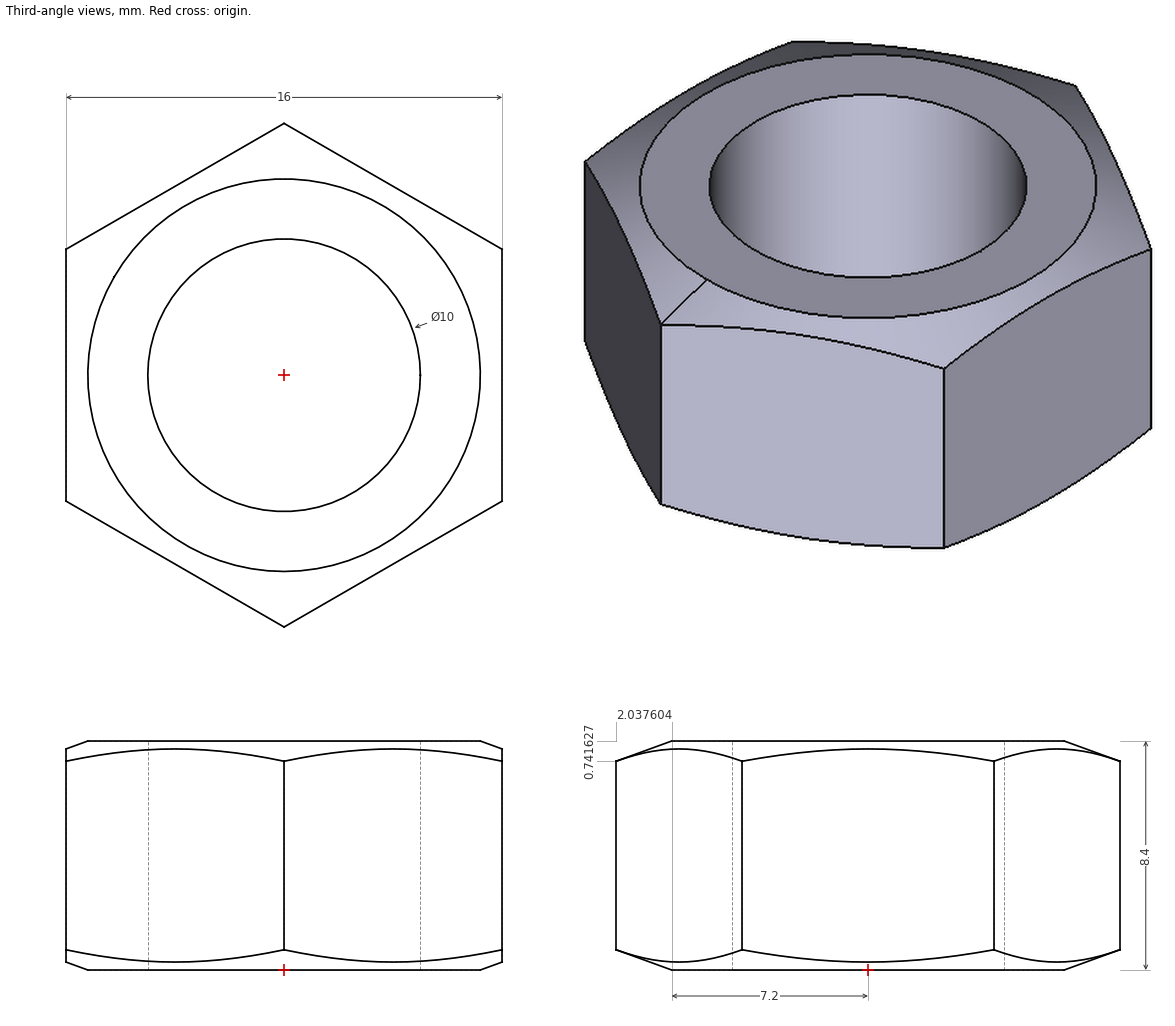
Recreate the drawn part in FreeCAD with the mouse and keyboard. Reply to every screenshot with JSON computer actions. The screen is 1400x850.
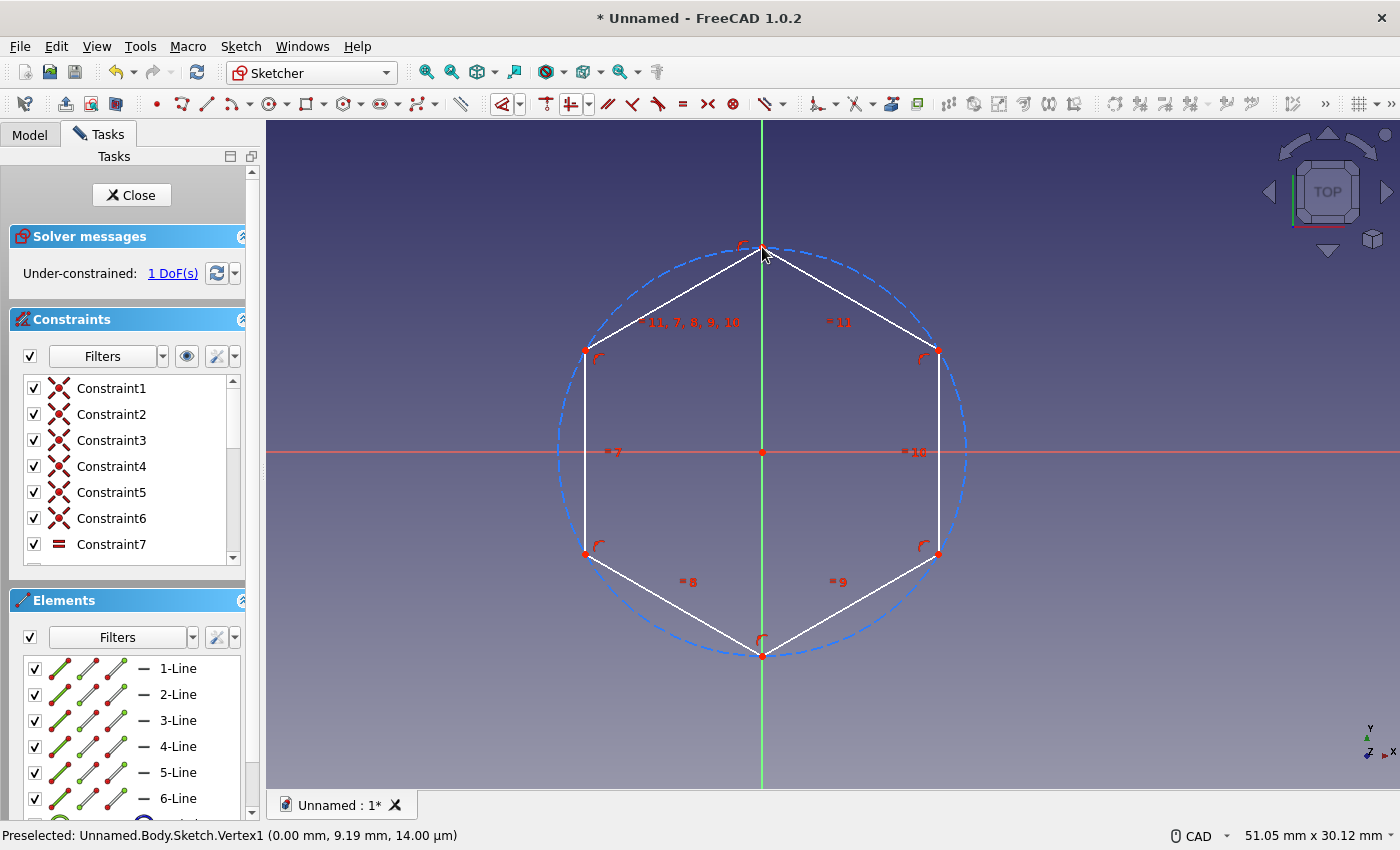
{"action": "left_click", "coordinate": [585, 350]}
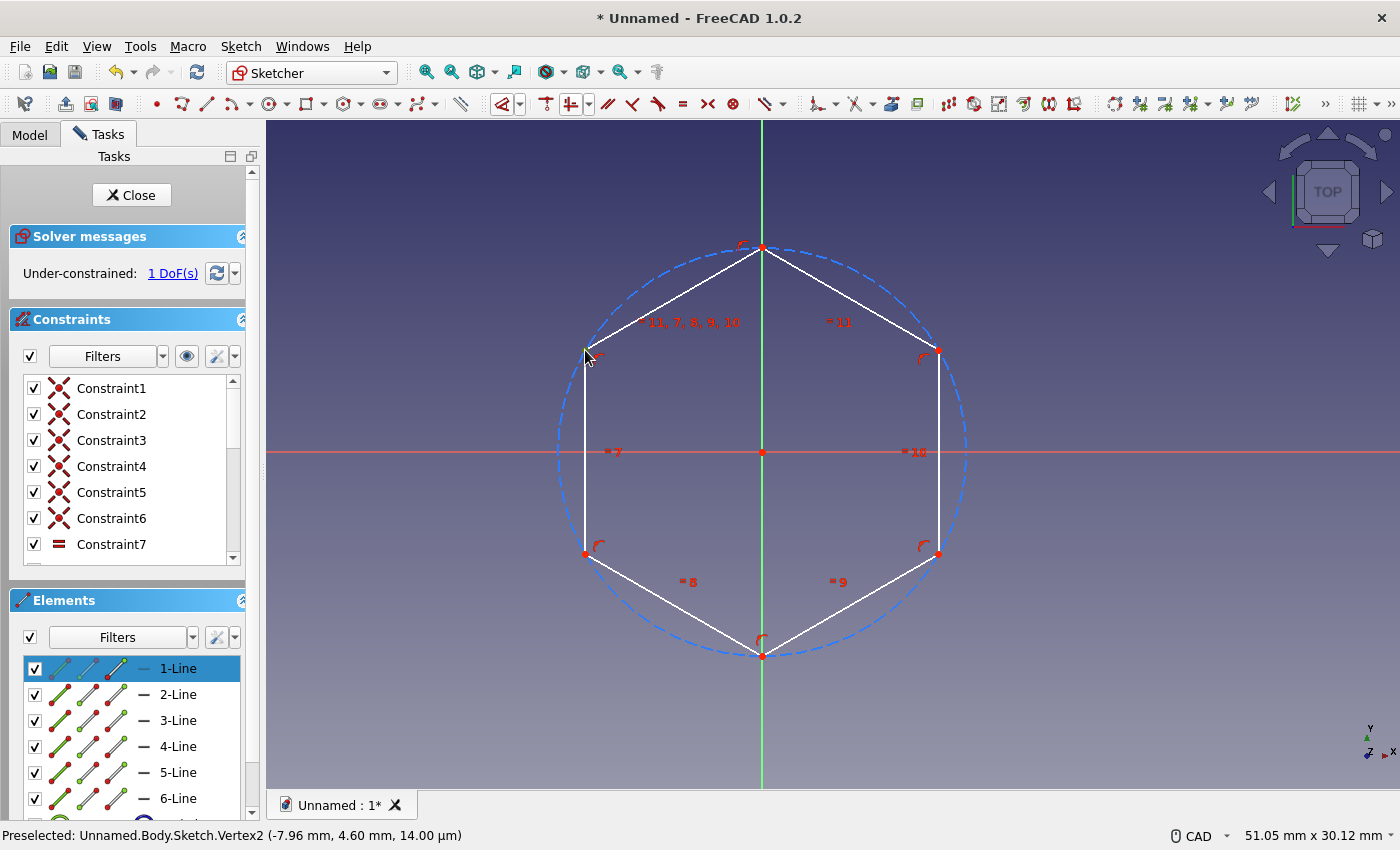
{"action": "left_click", "coordinate": [939, 554]}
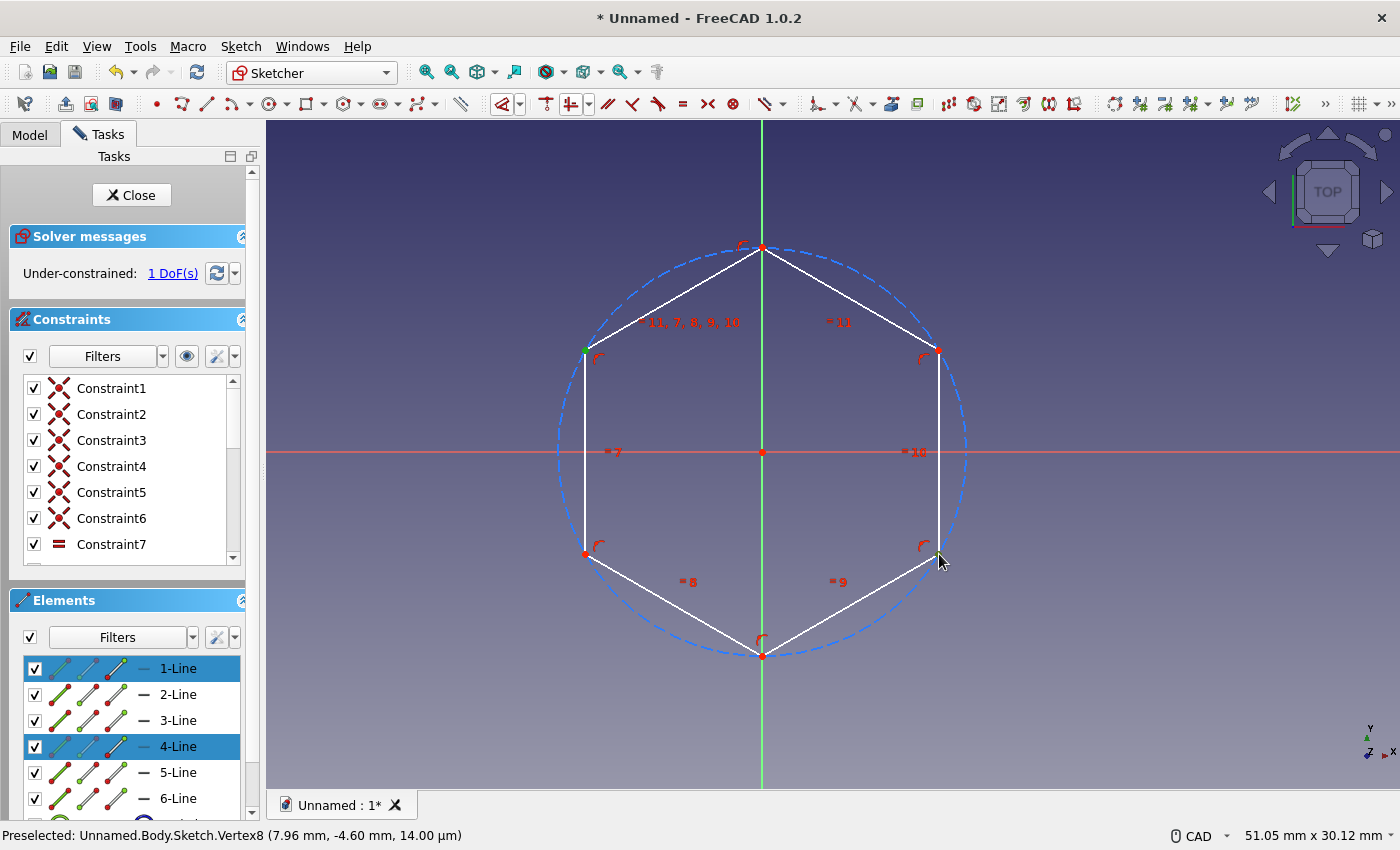
{"action": "left_click", "coordinate": [520, 104]}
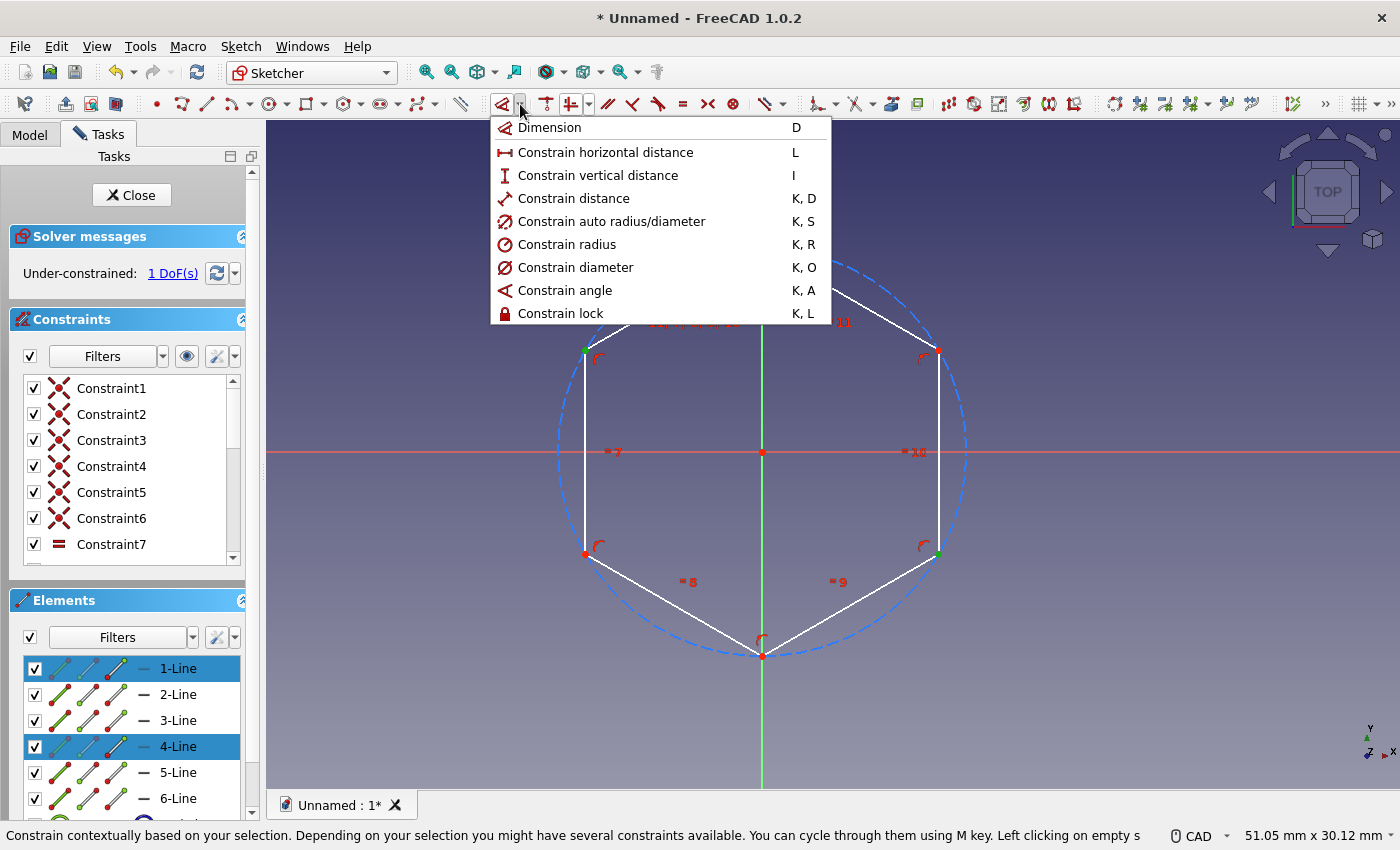
{"action": "left_click", "coordinate": [661, 152]}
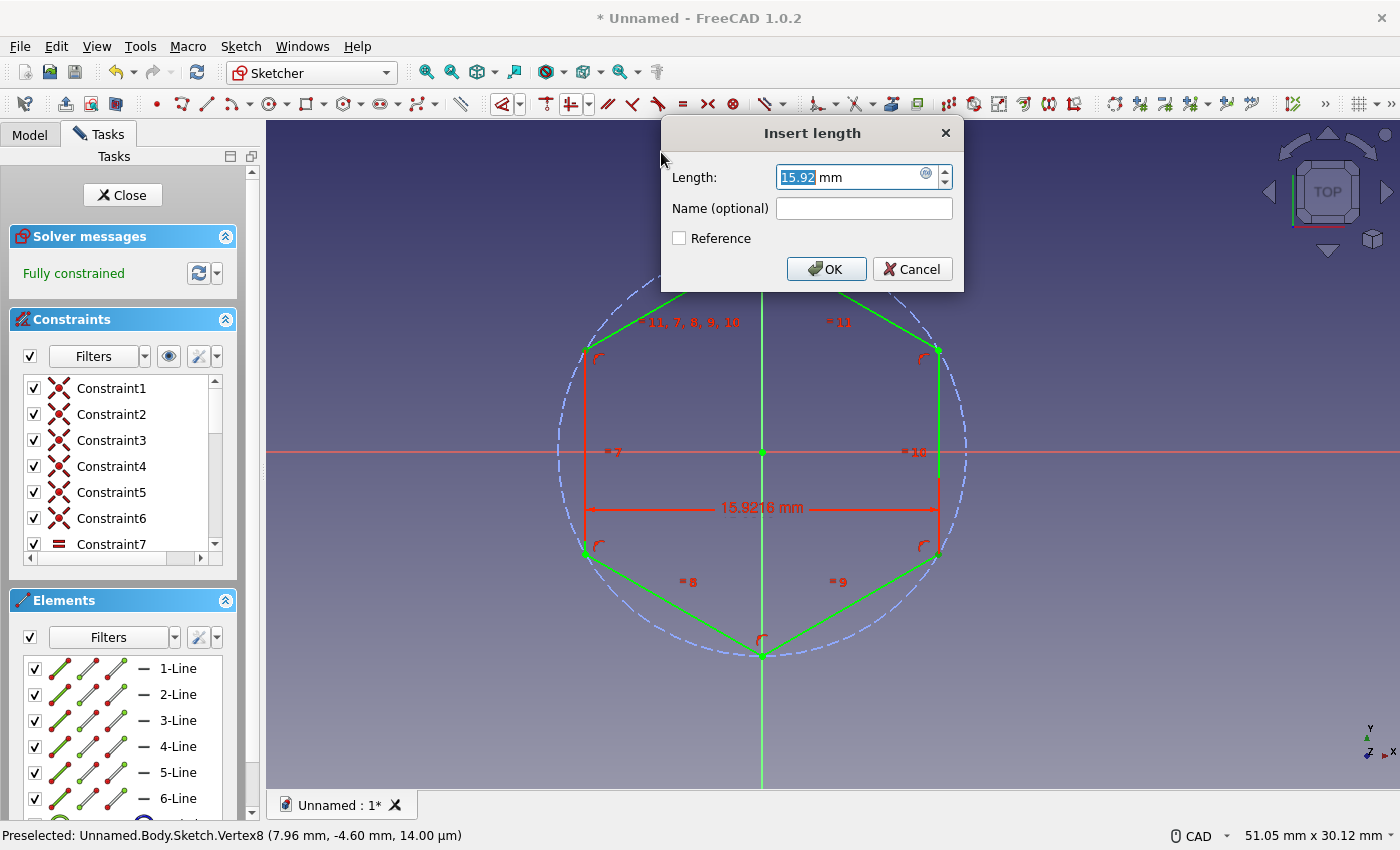
{"action": "type", "text": "16"}
{"action": "key", "text": "Return"}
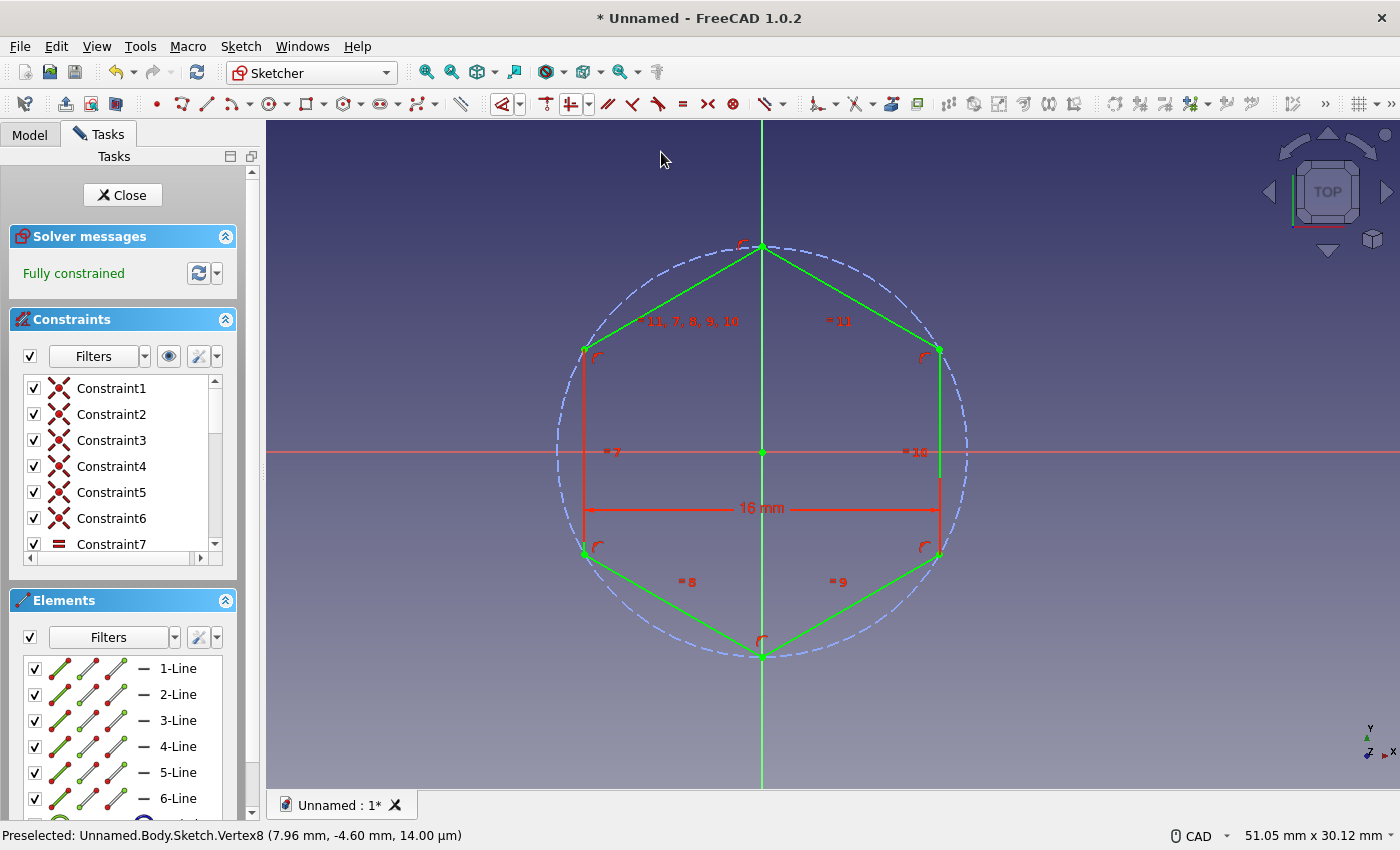
{"action": "left_click", "coordinate": [123, 195]}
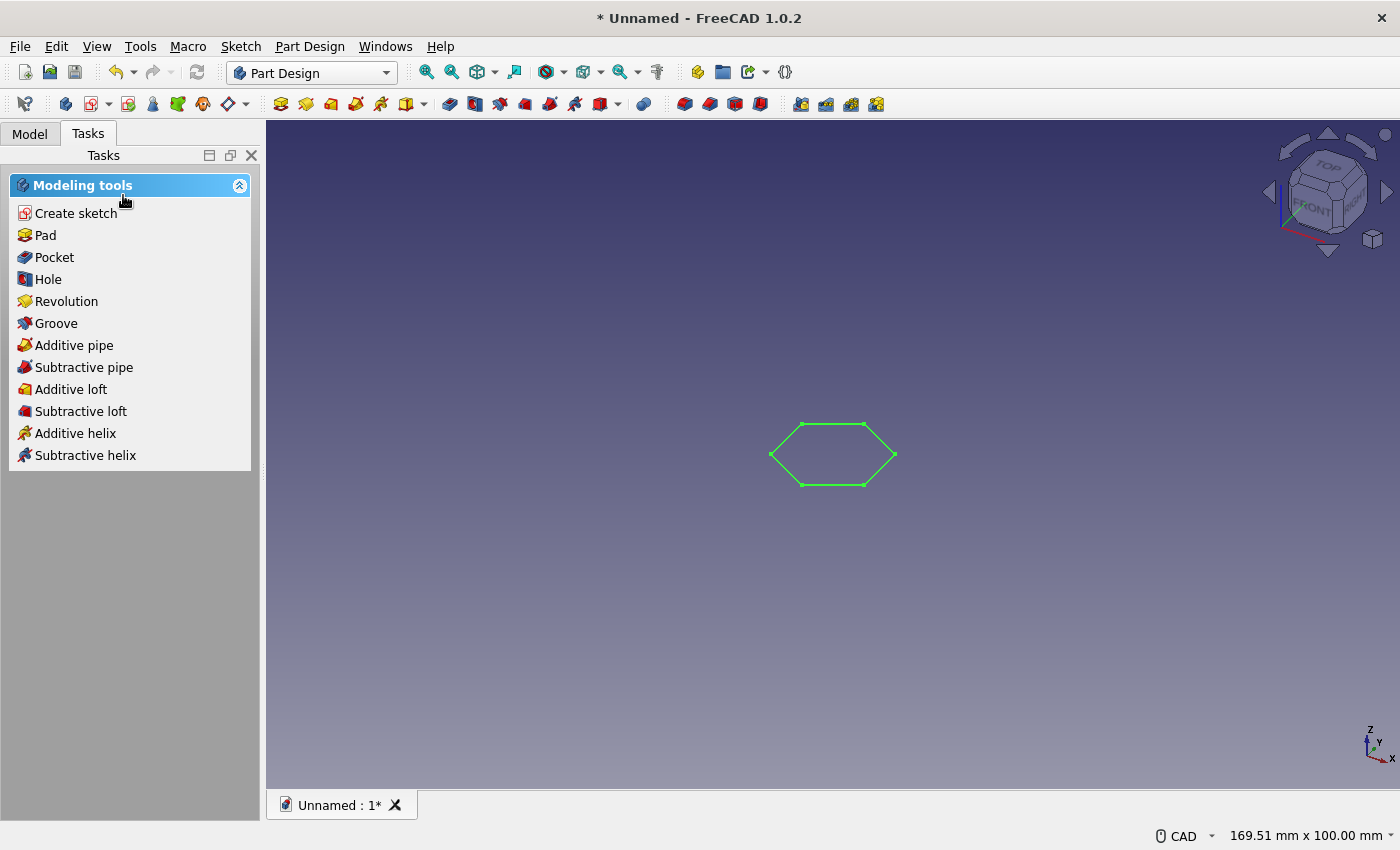
{"action": "left_click", "coordinate": [281, 104]}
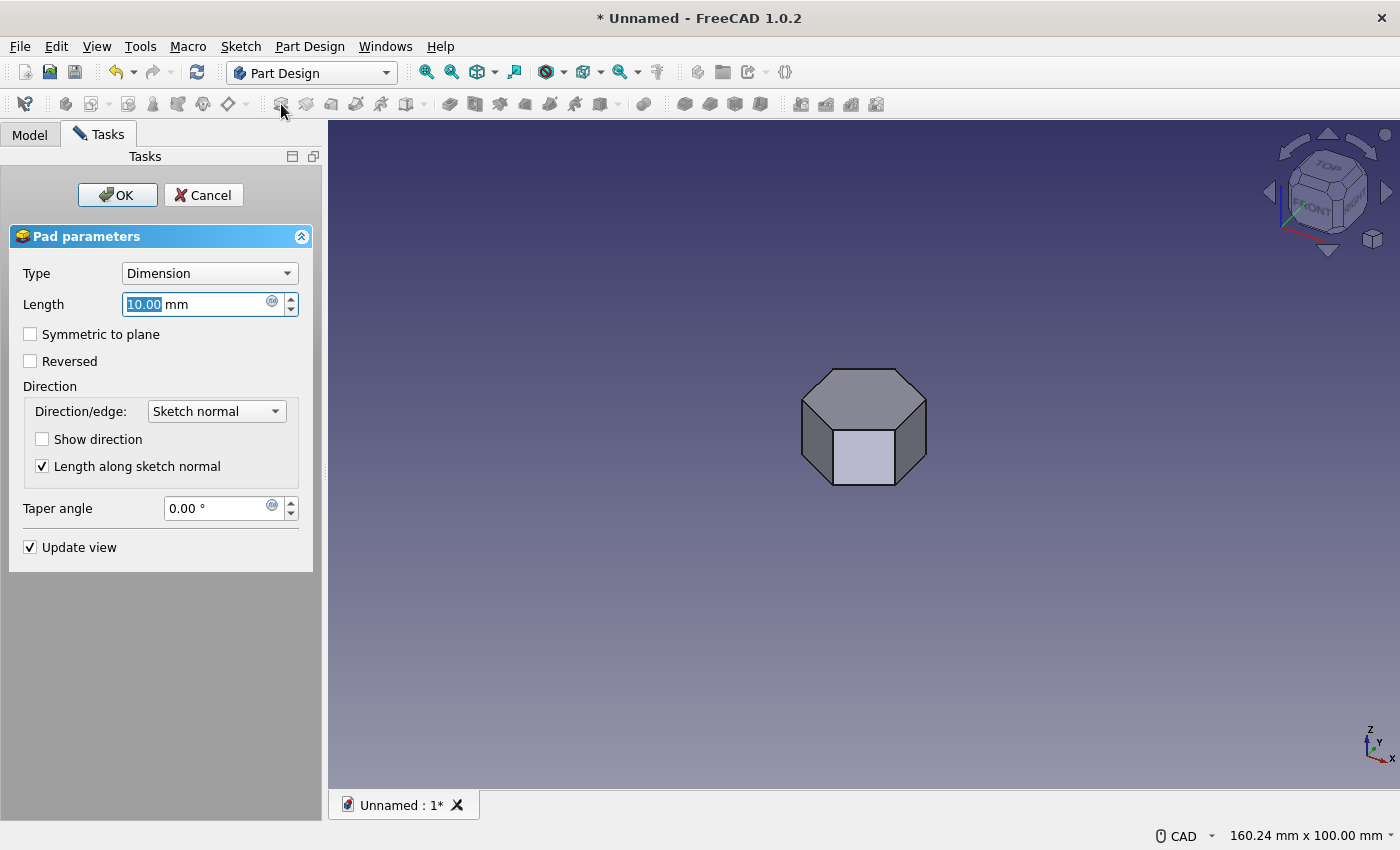
{"action": "type", "text": "8.4"}
{"action": "key", "text": "Tab"}